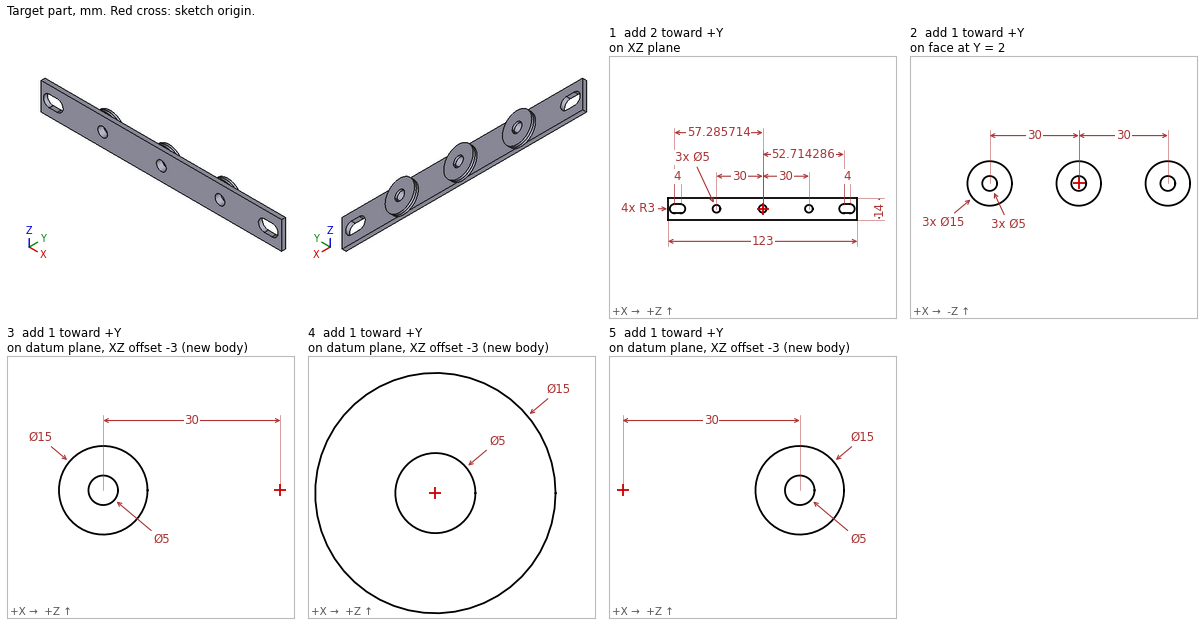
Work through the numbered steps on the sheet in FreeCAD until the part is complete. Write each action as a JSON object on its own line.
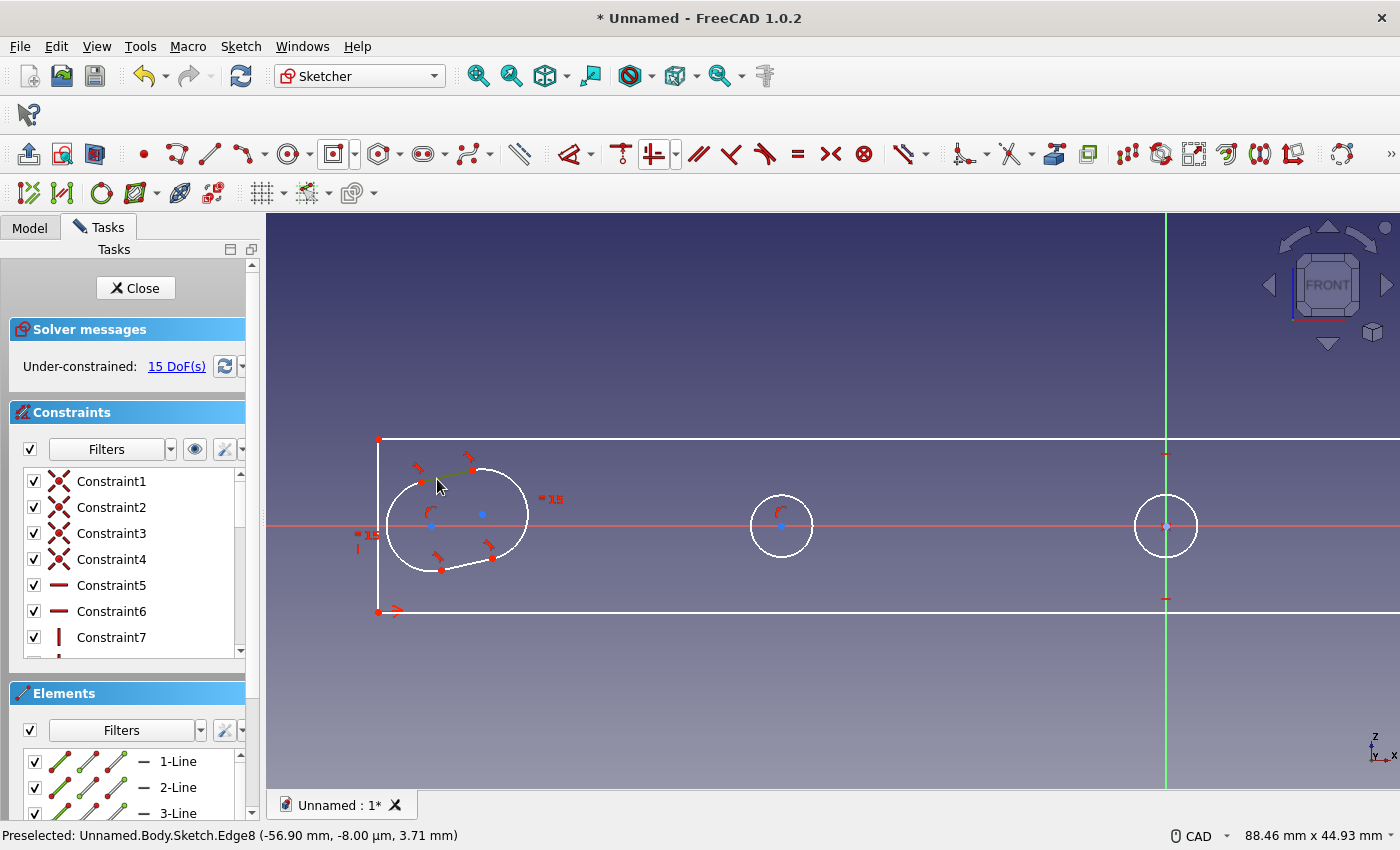
{"action": "key", "text": "h"}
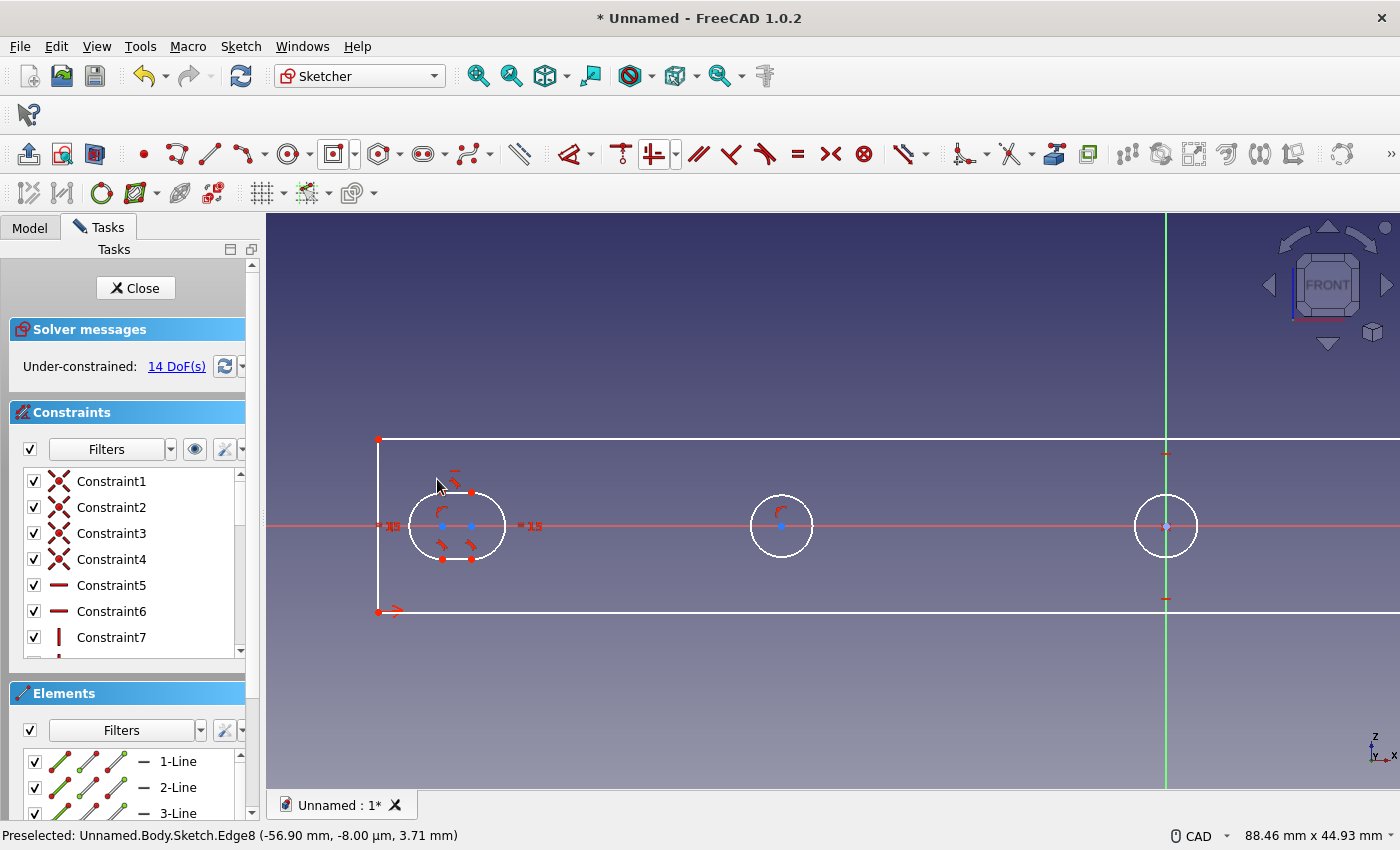
{"action": "scroll", "coordinate": [437, 480], "scroll_direction": "down", "scroll_amount": 4}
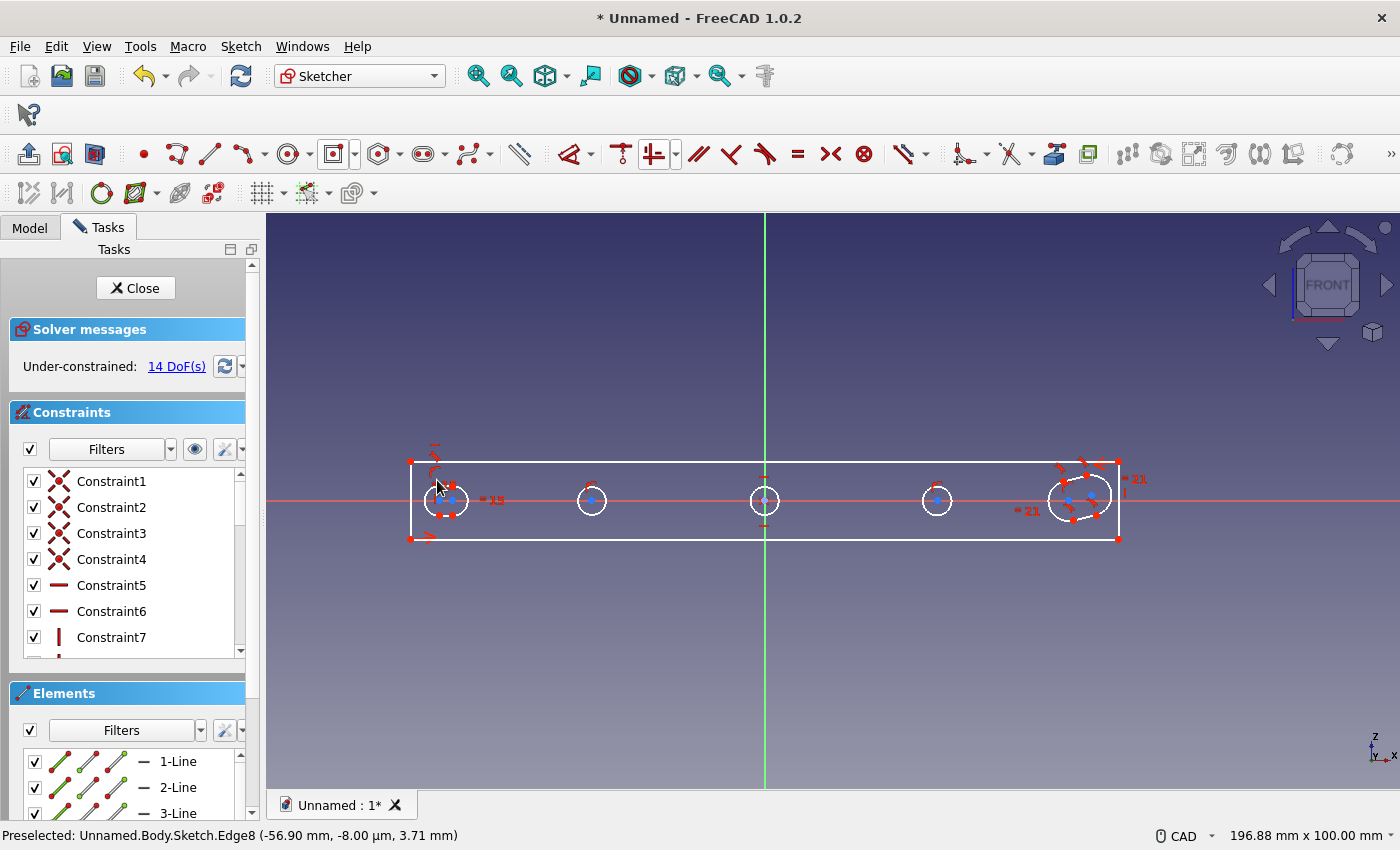
{"action": "scroll", "coordinate": [1071, 480], "scroll_direction": "up", "scroll_amount": 4}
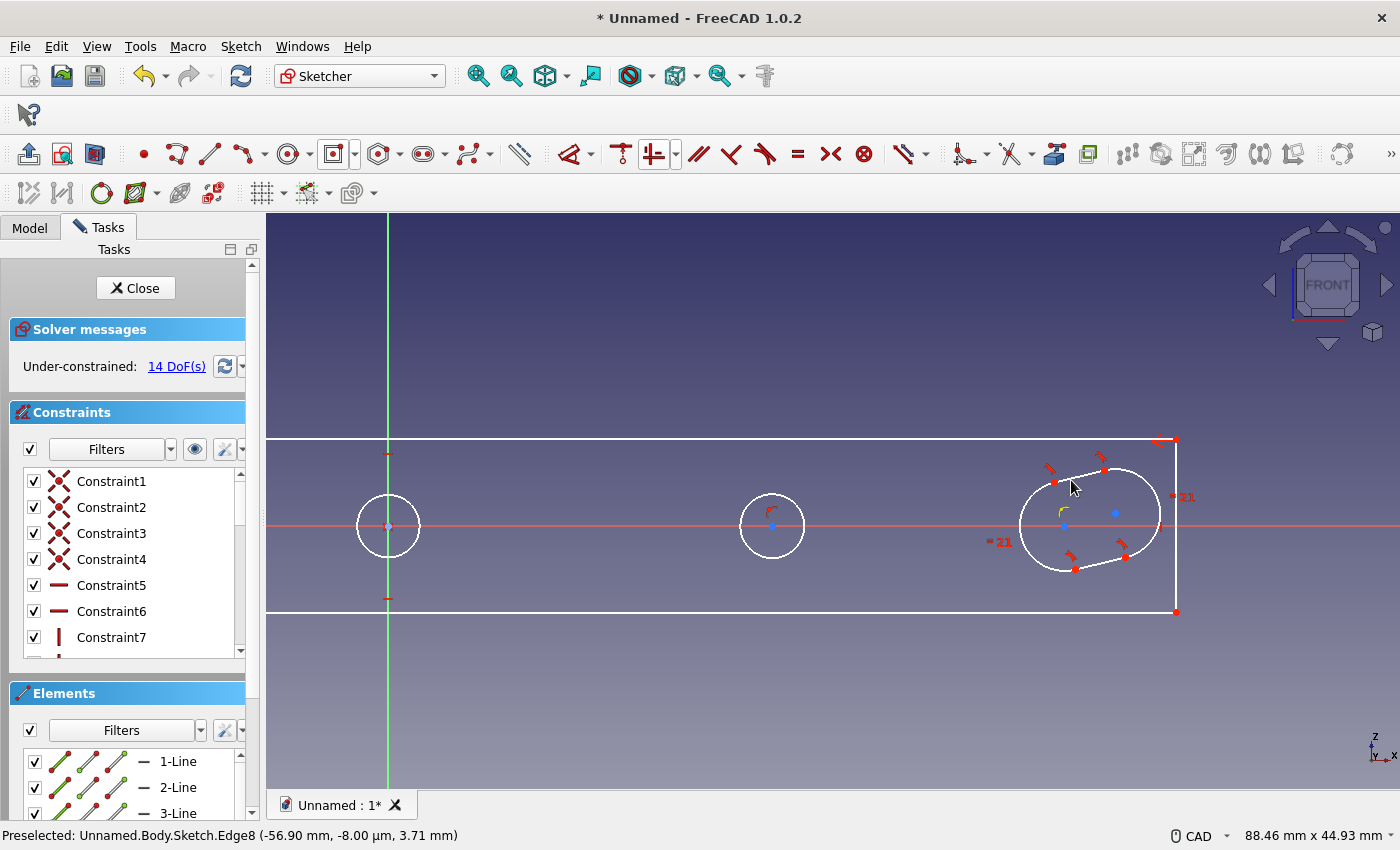
{"action": "left_click", "coordinate": [1069, 479]}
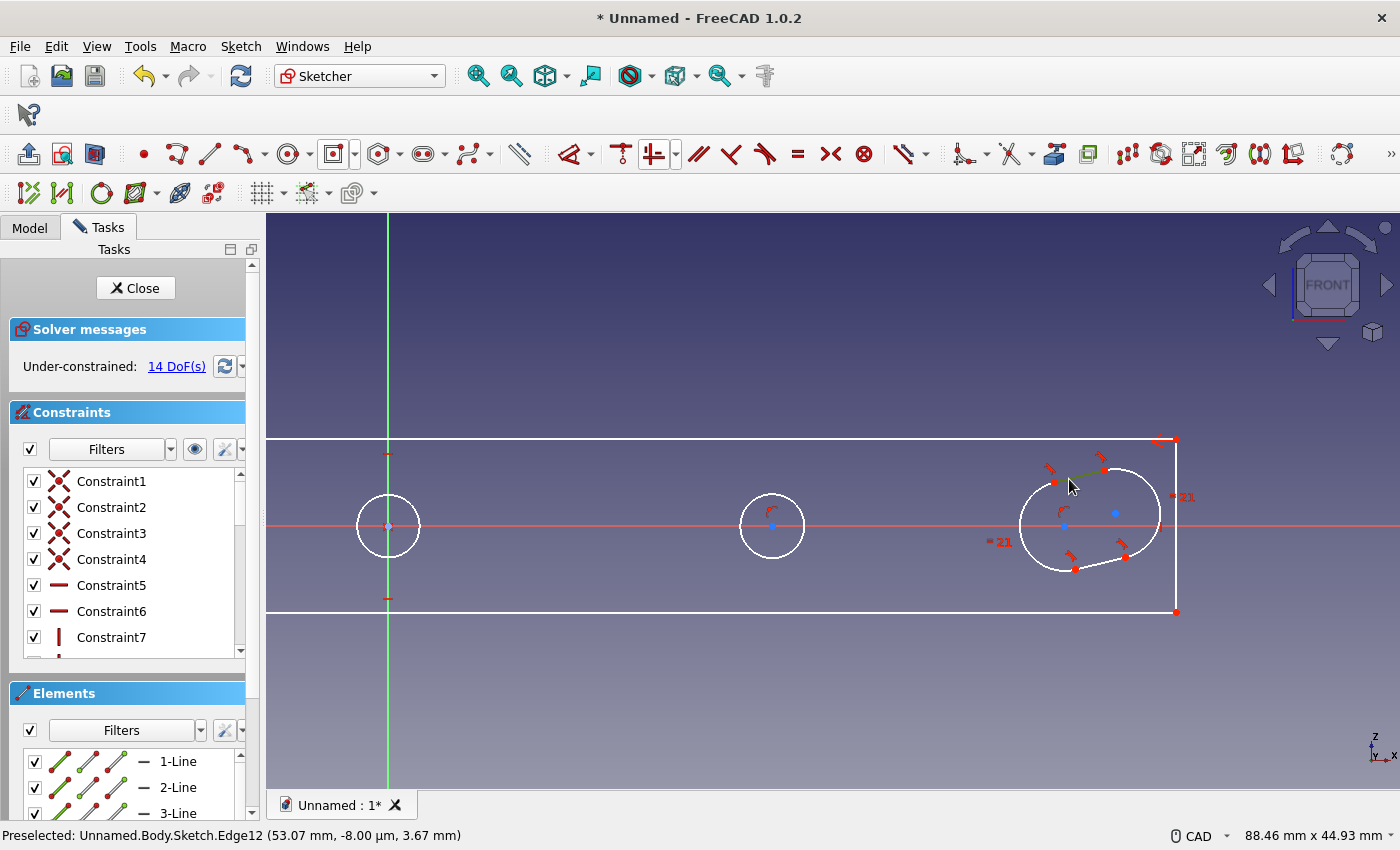
{"action": "key", "text": "h"}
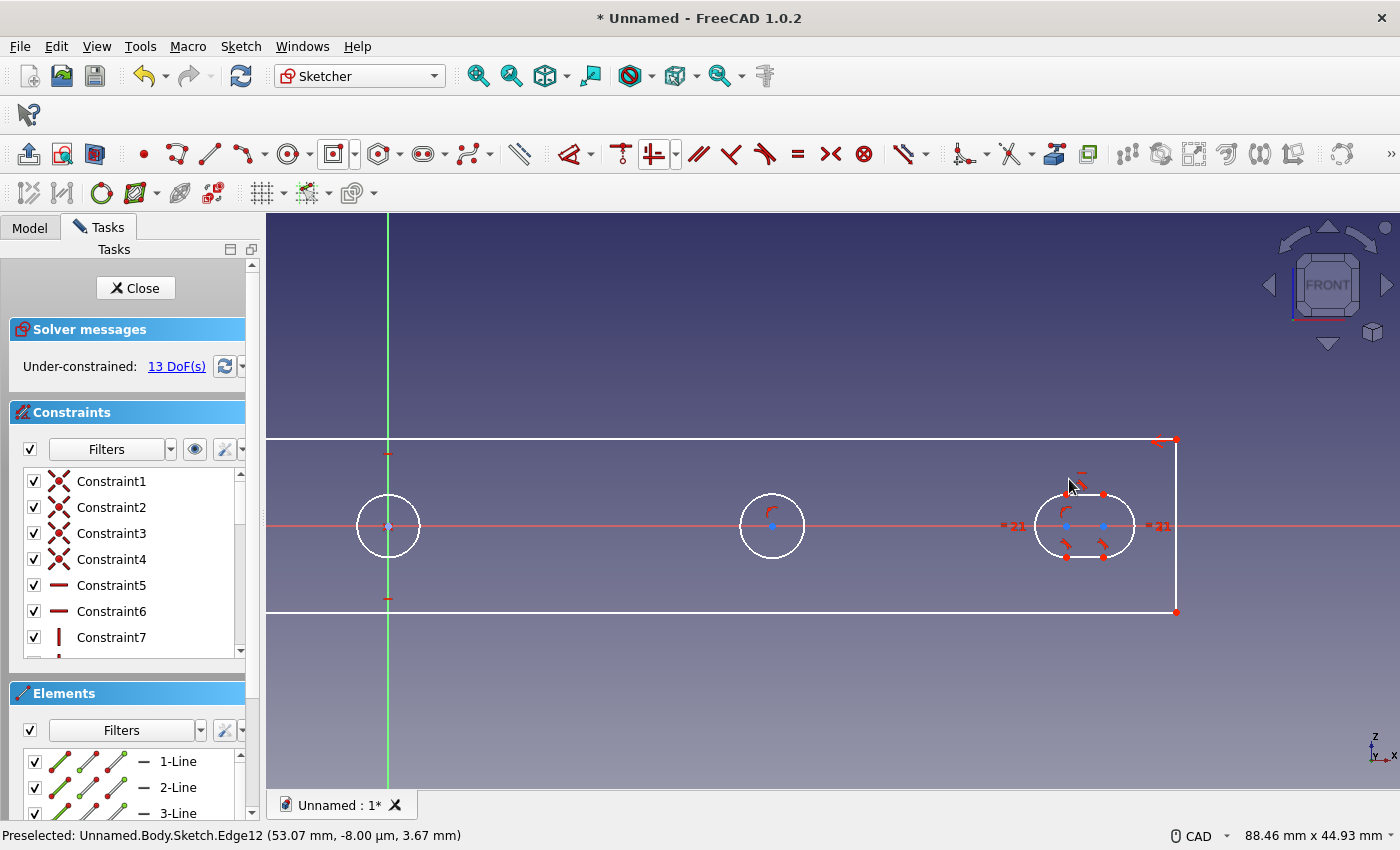
{"action": "scroll", "coordinate": [1071, 480], "scroll_direction": "down", "scroll_amount": 4}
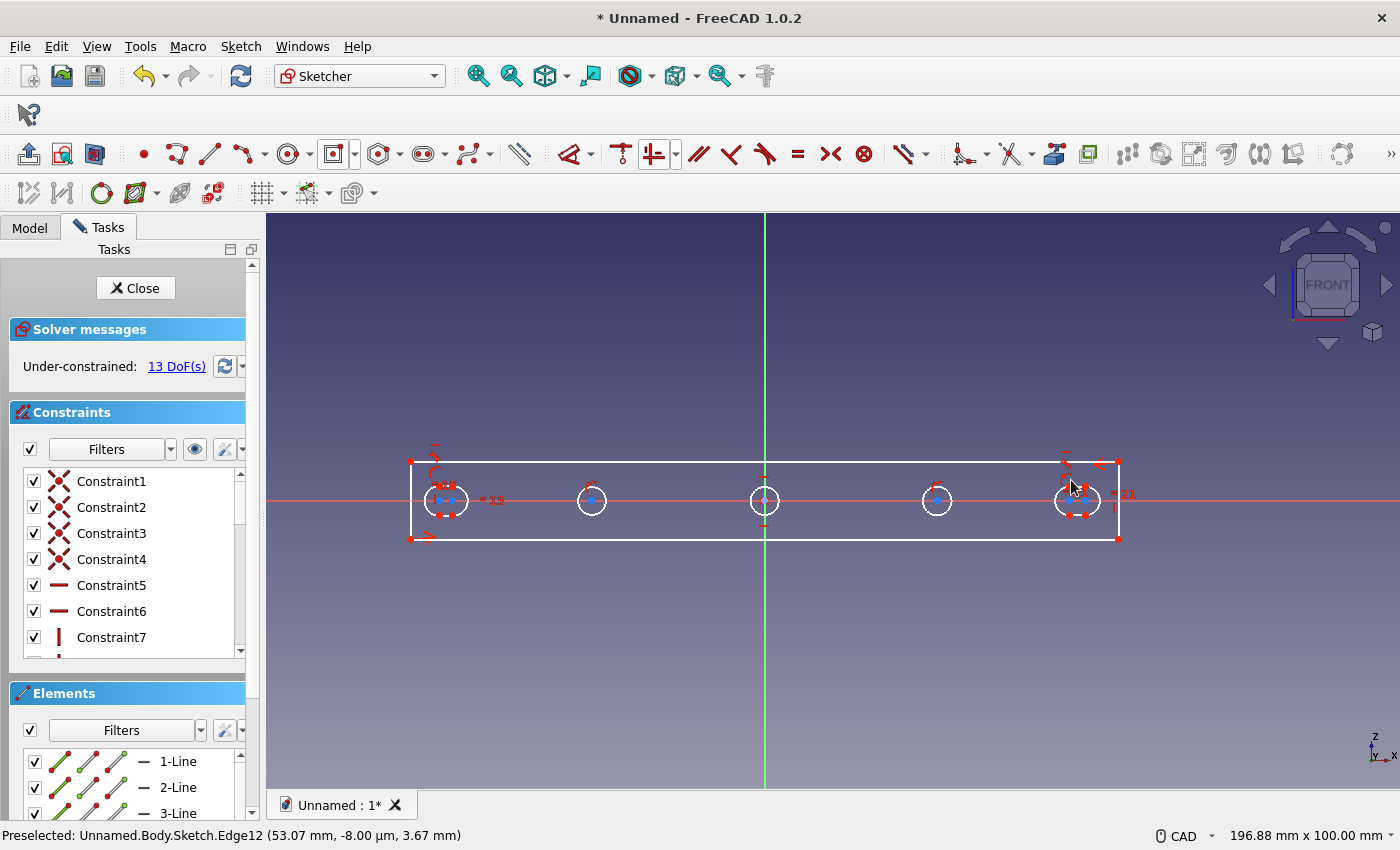
{"action": "scroll", "coordinate": [427, 492], "scroll_direction": "up", "scroll_amount": 3}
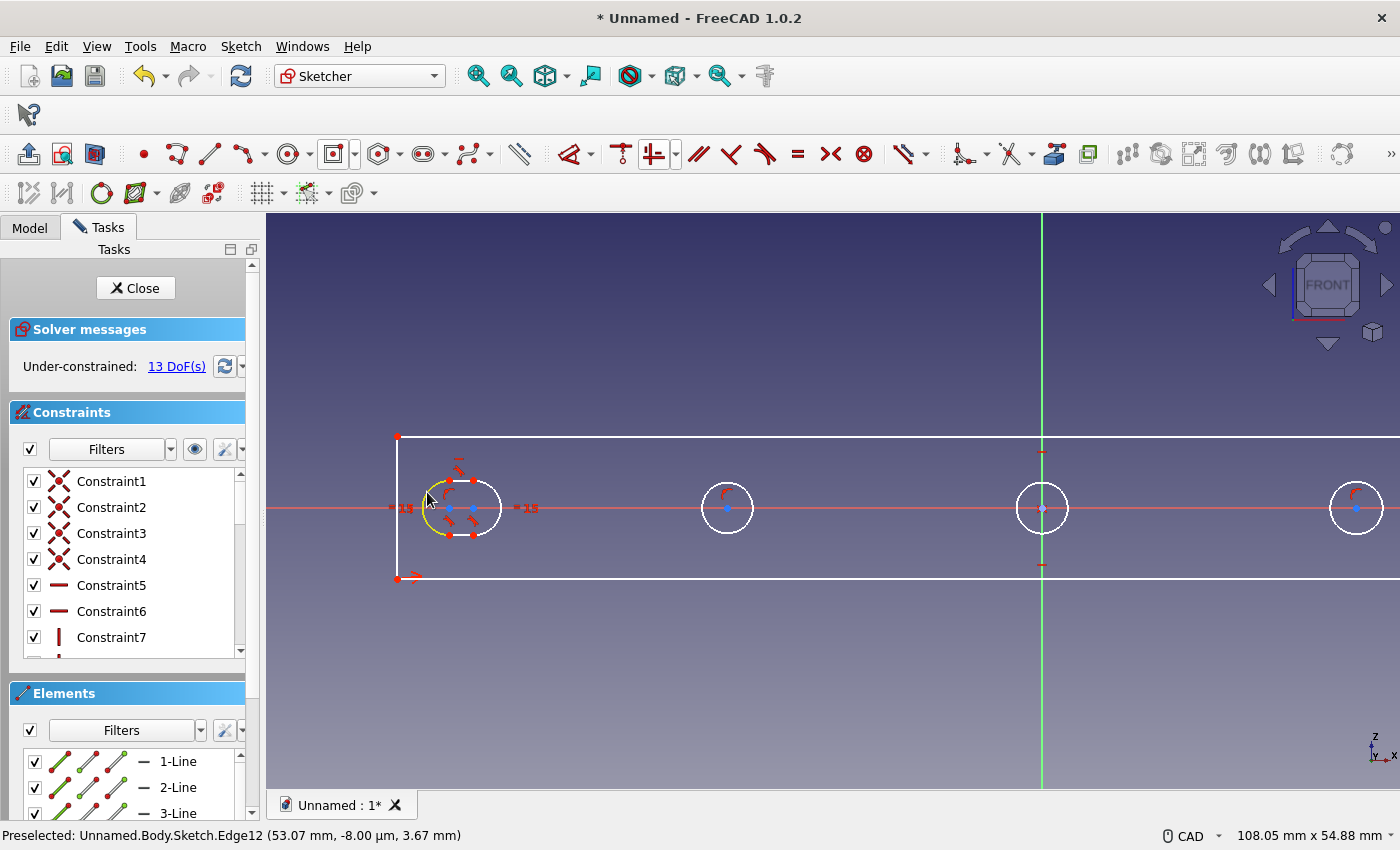
{"action": "left_click", "coordinate": [428, 492]}